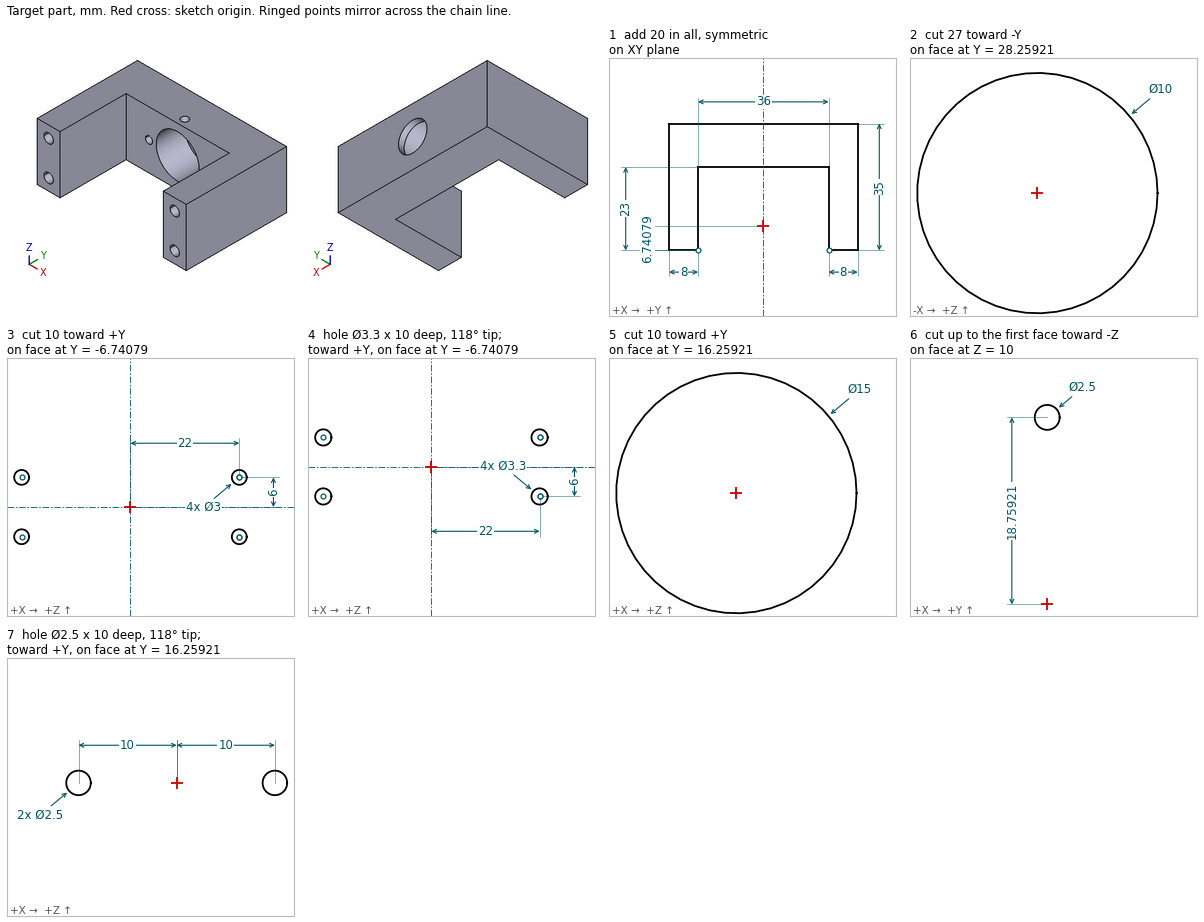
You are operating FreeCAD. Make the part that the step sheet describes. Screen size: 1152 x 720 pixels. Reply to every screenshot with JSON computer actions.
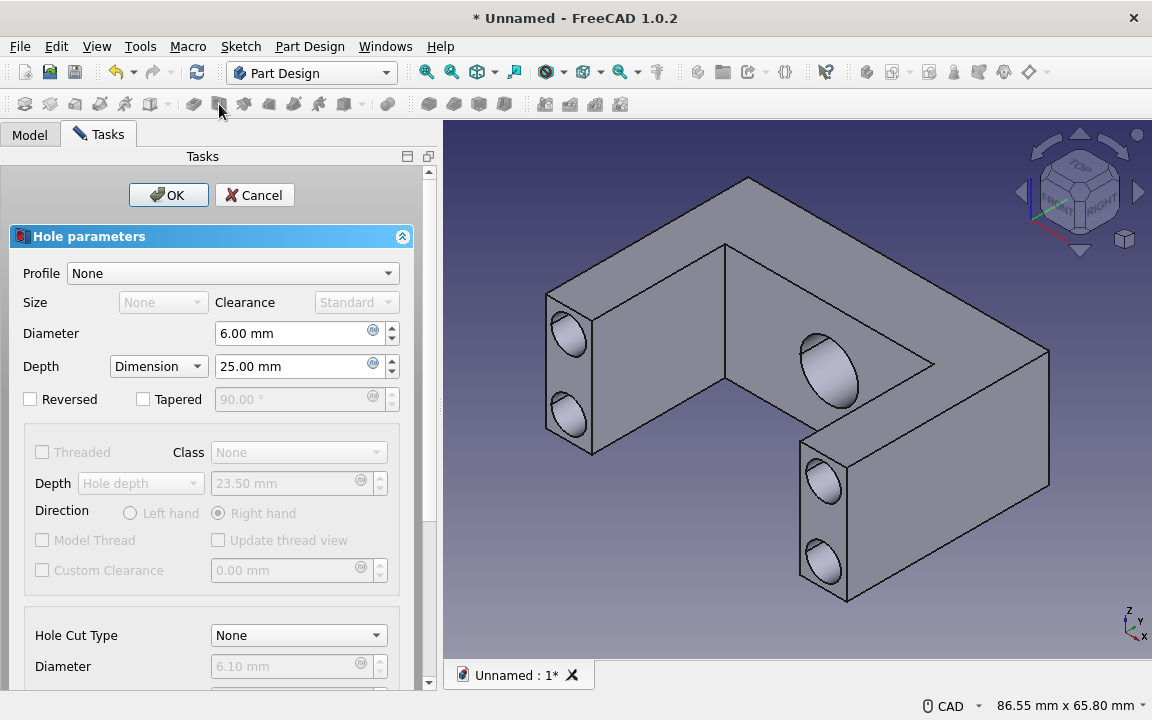
{"action": "triple_click", "coordinate": [300, 334]}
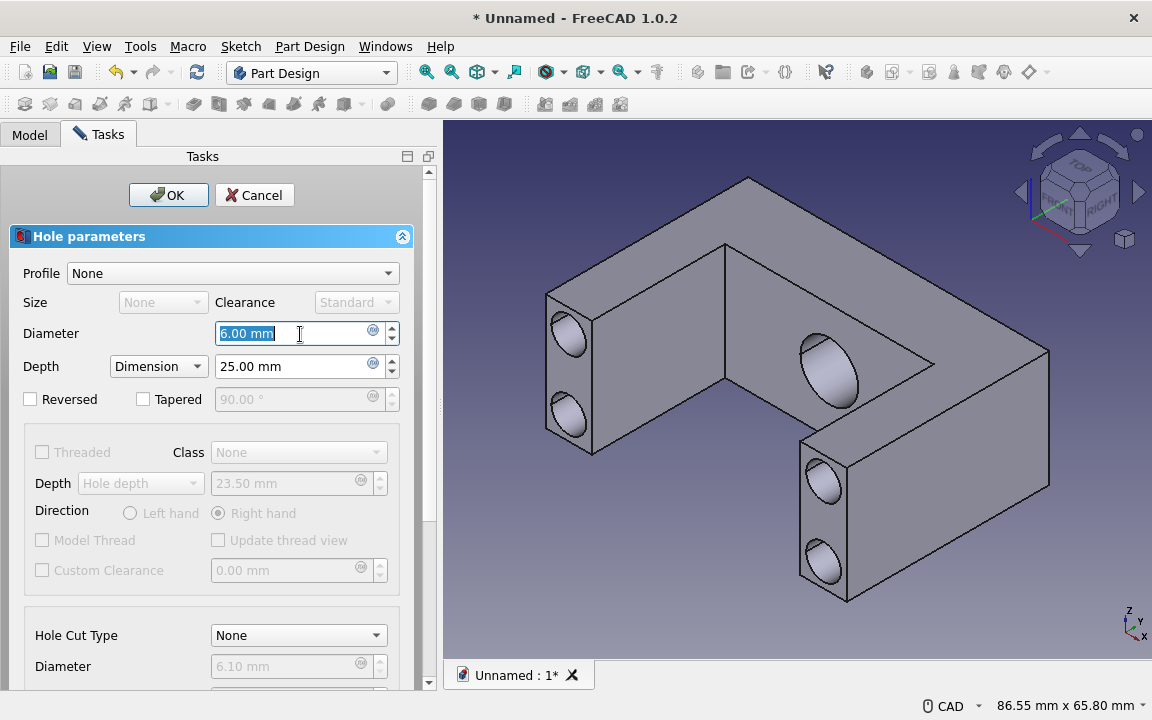
{"action": "type", "text": "3.3"}
{"action": "key", "text": "Tab"}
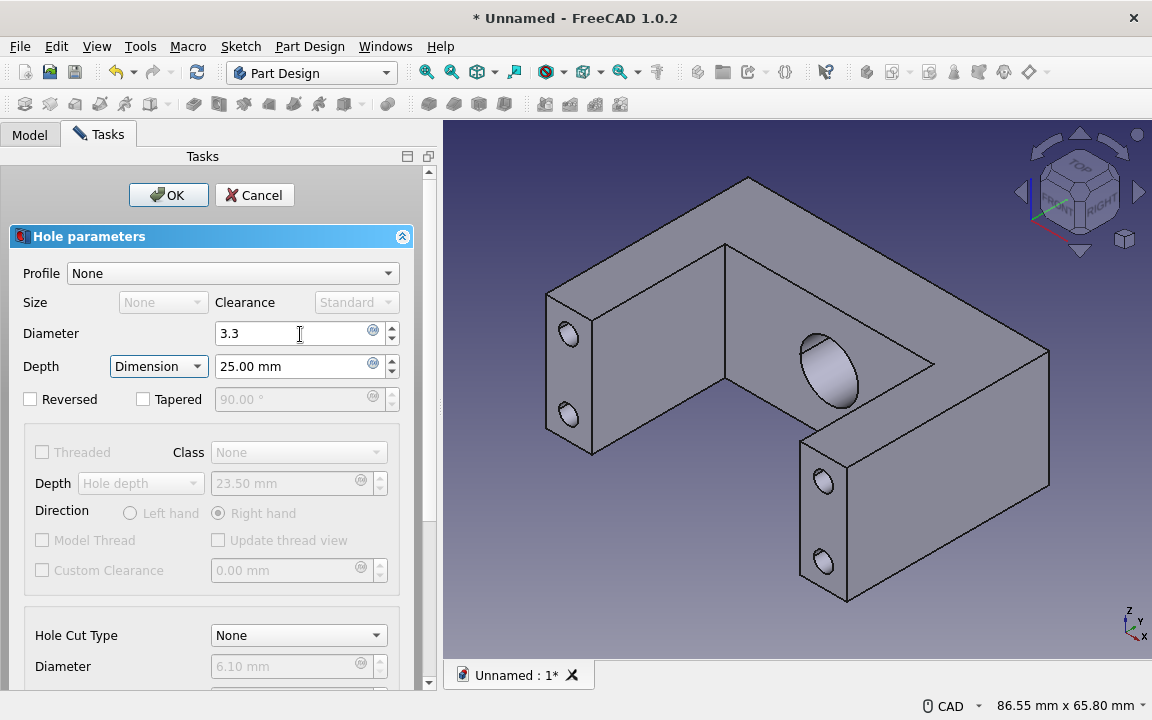
{"action": "triple_click", "coordinate": [300, 366]}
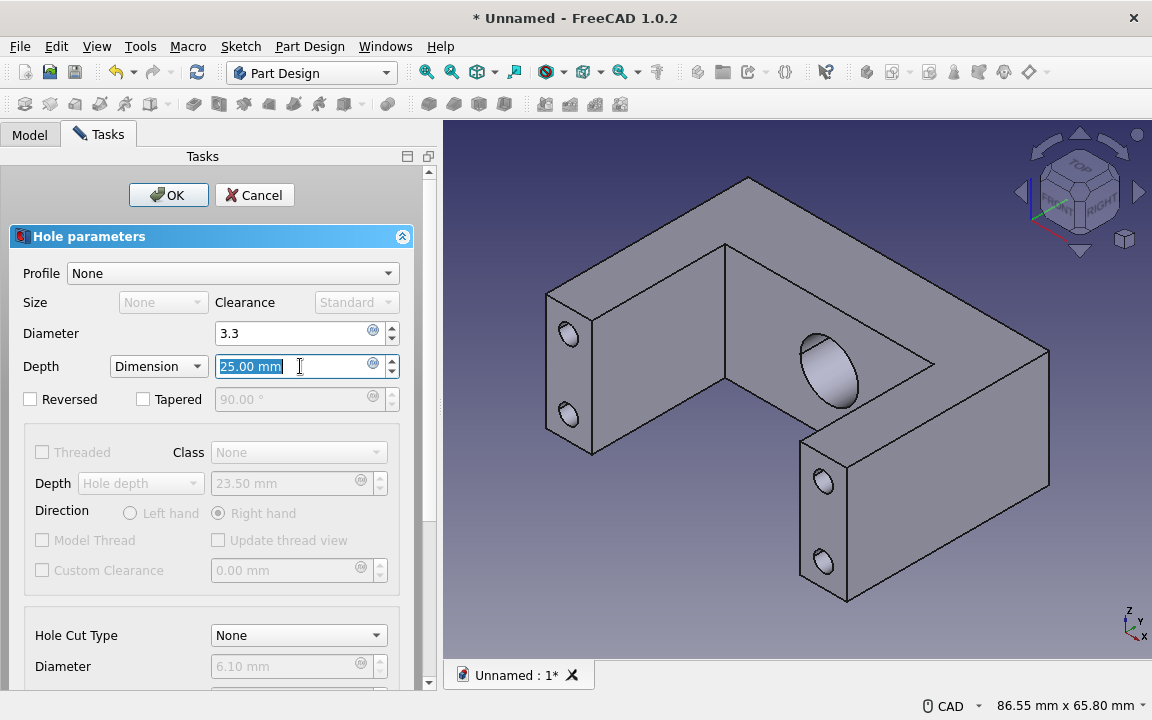
{"action": "type", "text": "10"}
{"action": "key", "text": "Tab"}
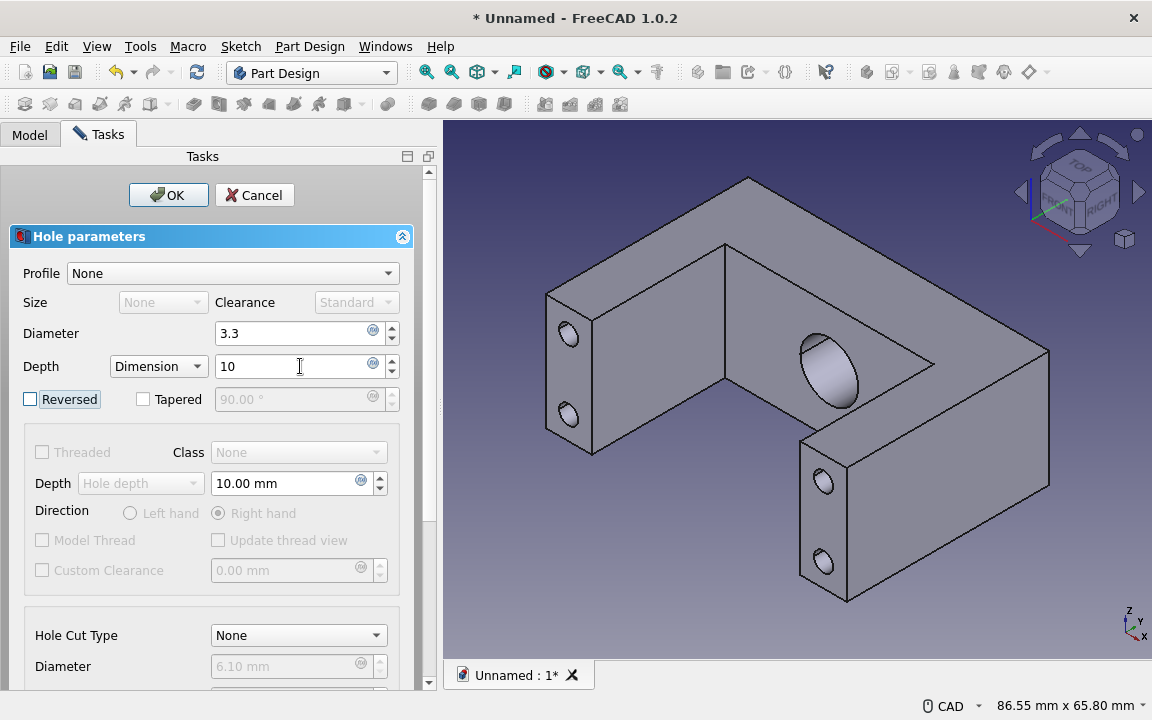
{"action": "left_click", "coordinate": [169, 195]}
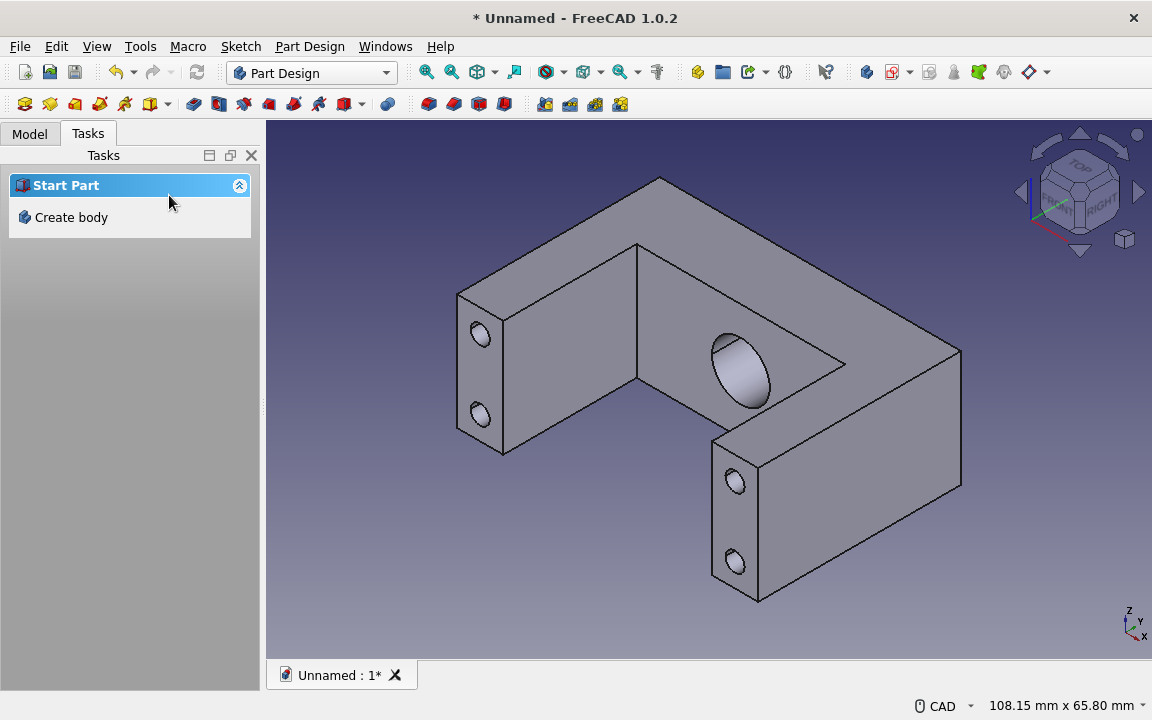
{"action": "left_click", "coordinate": [681, 355]}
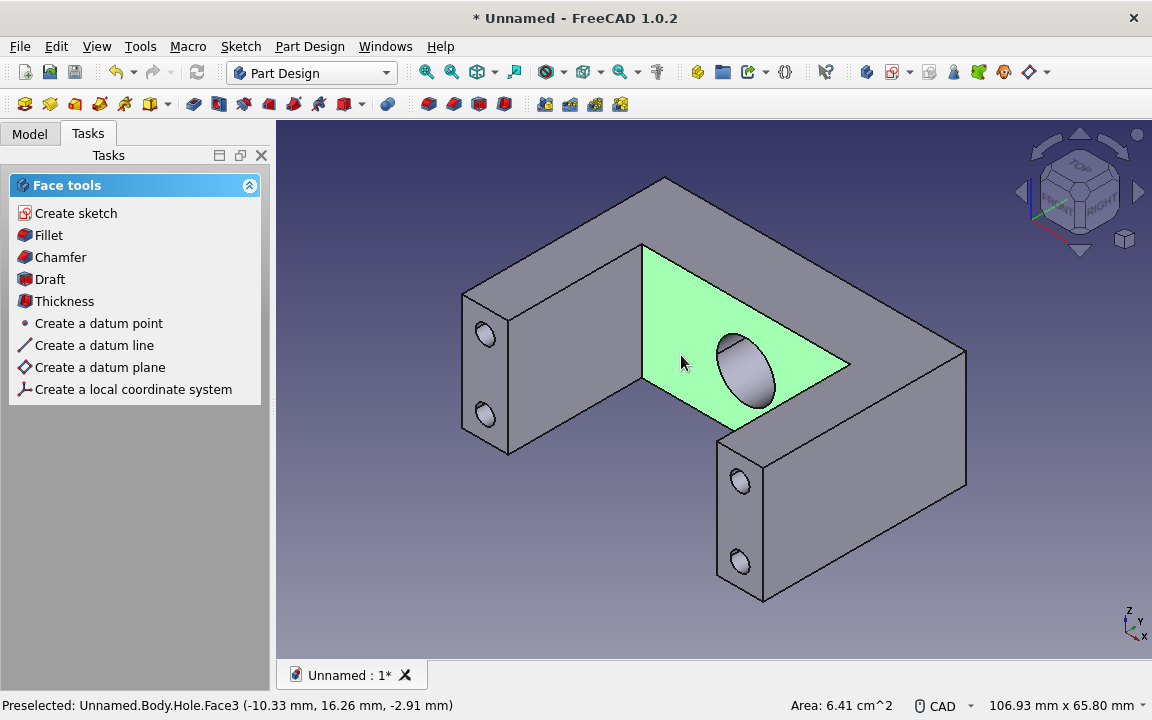
{"action": "left_click", "coordinate": [892, 72]}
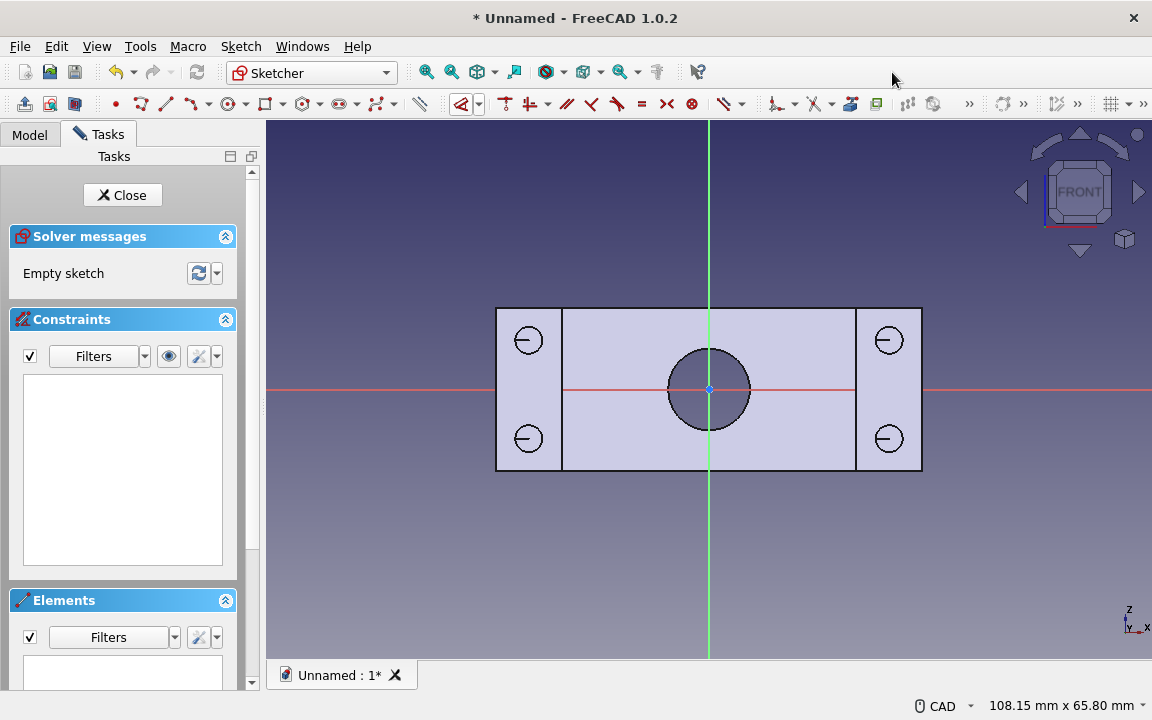
{"action": "scroll", "coordinate": [749, 390], "scroll_direction": "up", "scroll_amount": 5}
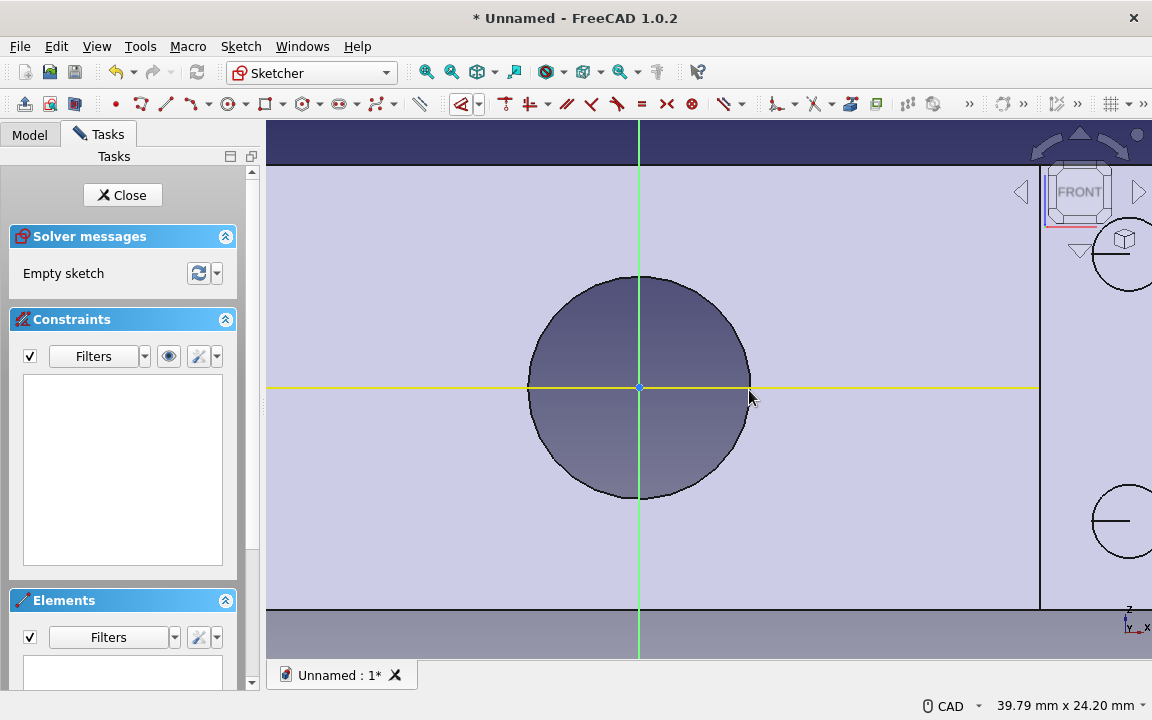
{"action": "left_click", "coordinate": [228, 104]}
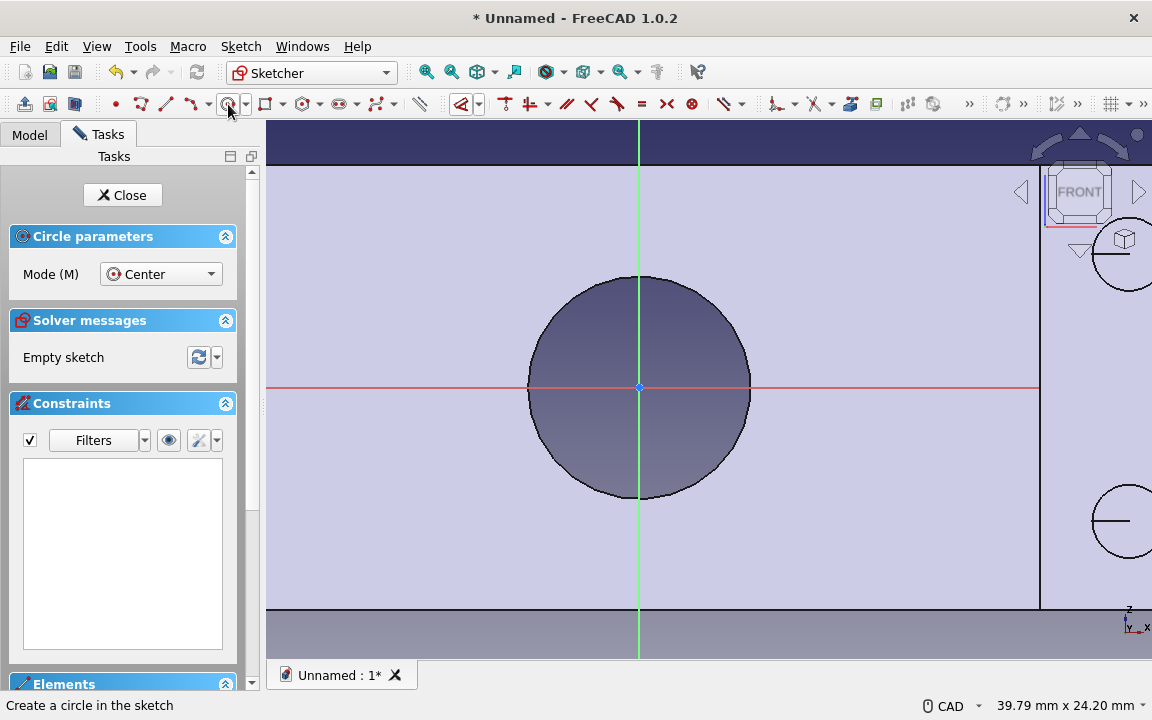
{"action": "left_click", "coordinate": [639, 388]}
{"action": "left_click", "coordinate": [757, 270]}
{"action": "key", "text": "Escape"}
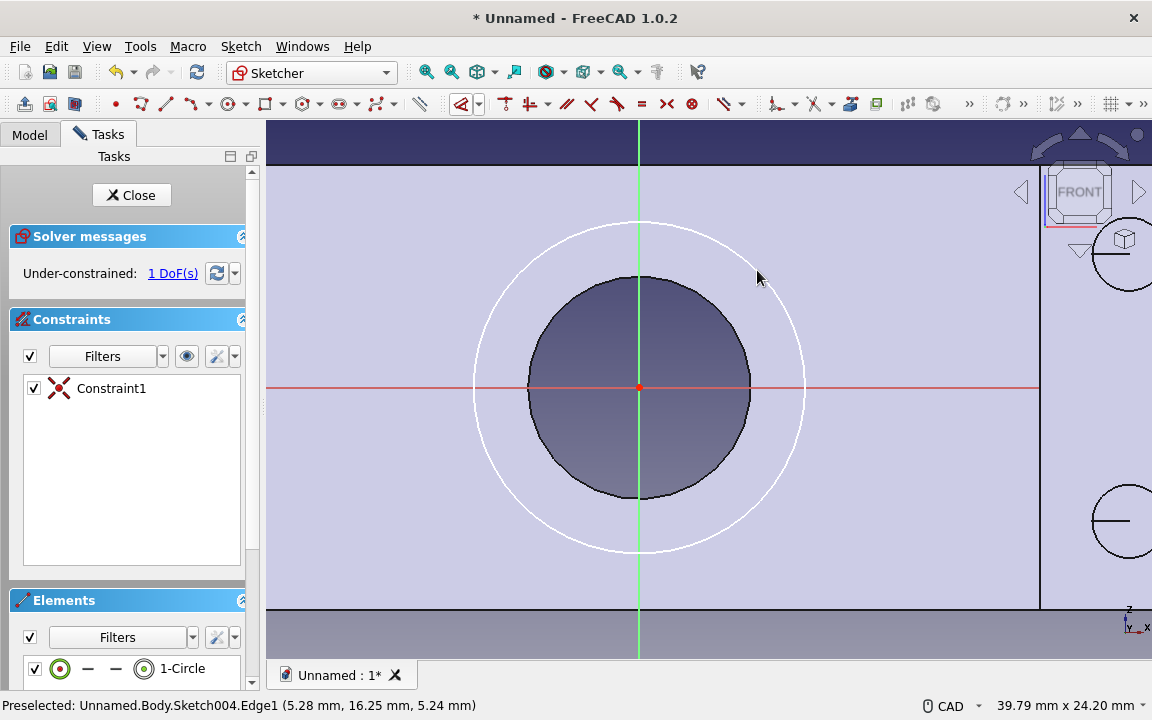
{"action": "left_click", "coordinate": [756, 270]}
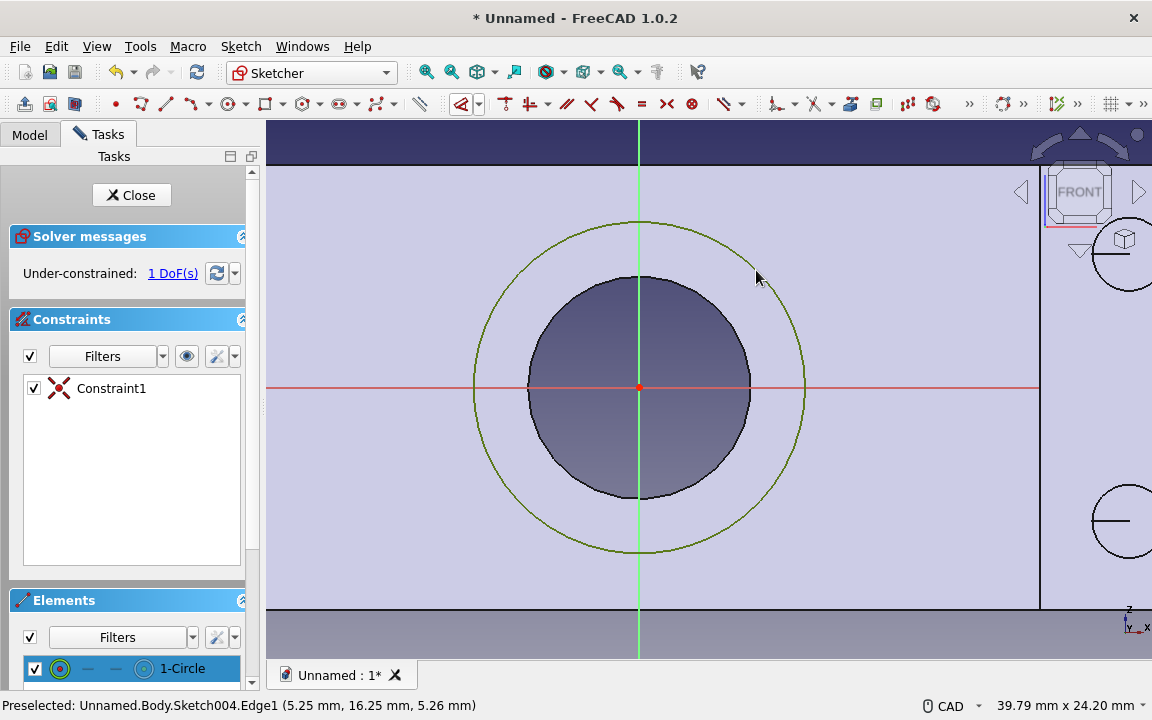
{"action": "key", "text": "k o"}